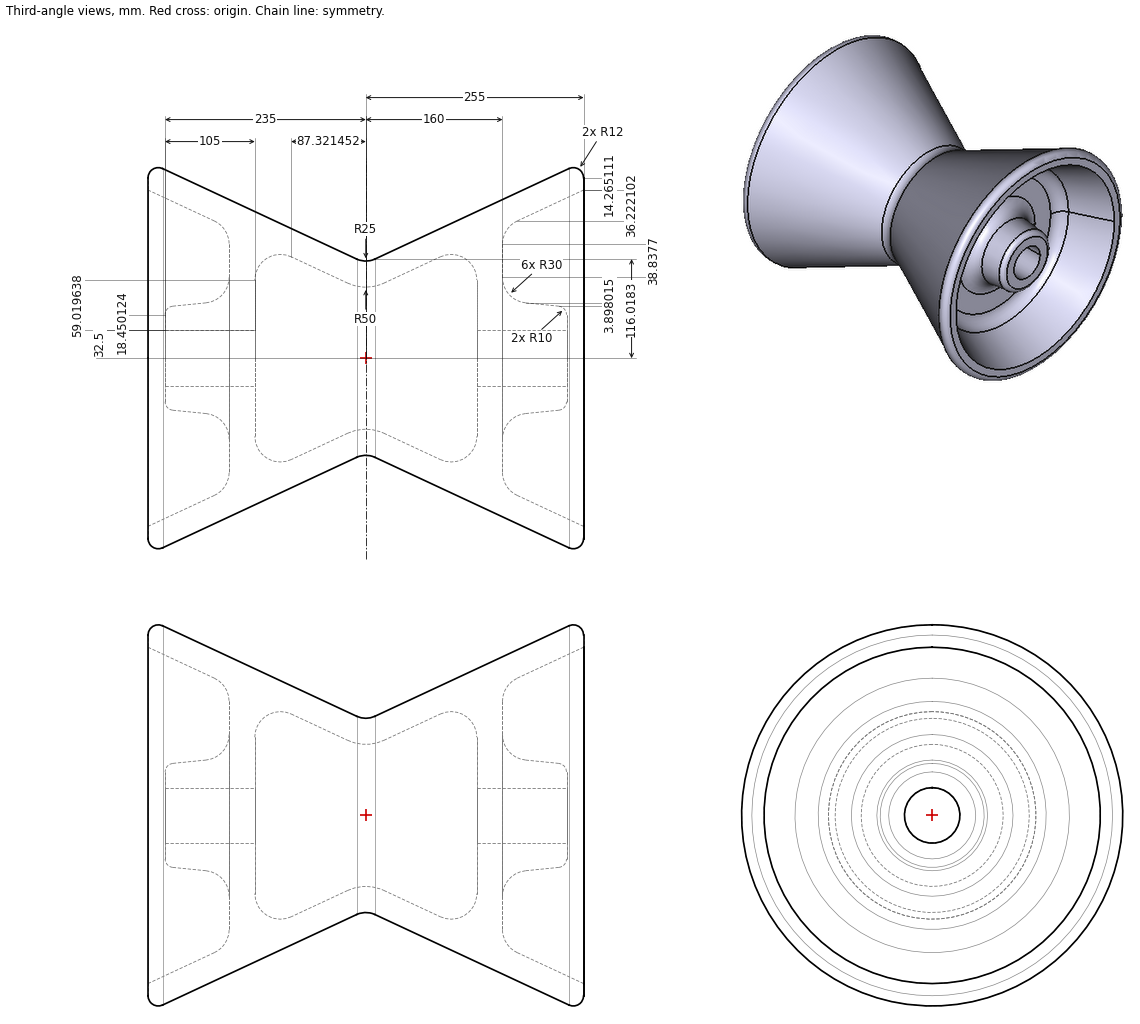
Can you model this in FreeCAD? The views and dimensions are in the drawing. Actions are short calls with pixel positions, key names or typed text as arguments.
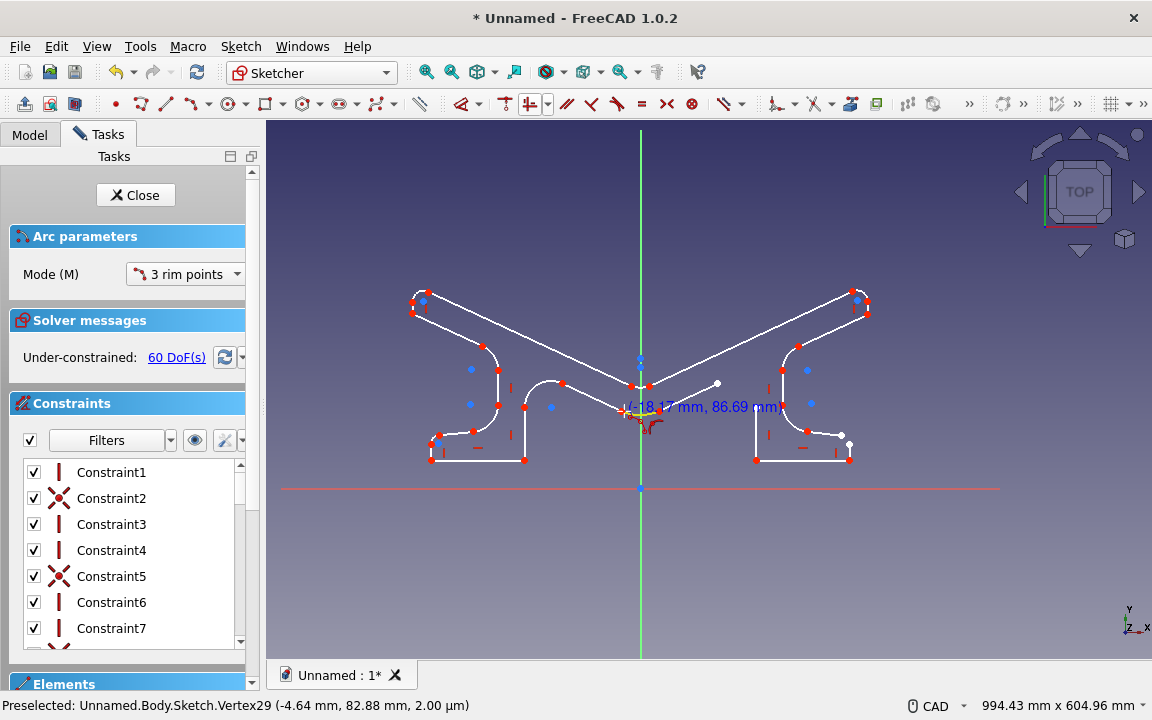
click(718, 384)
click(756, 408)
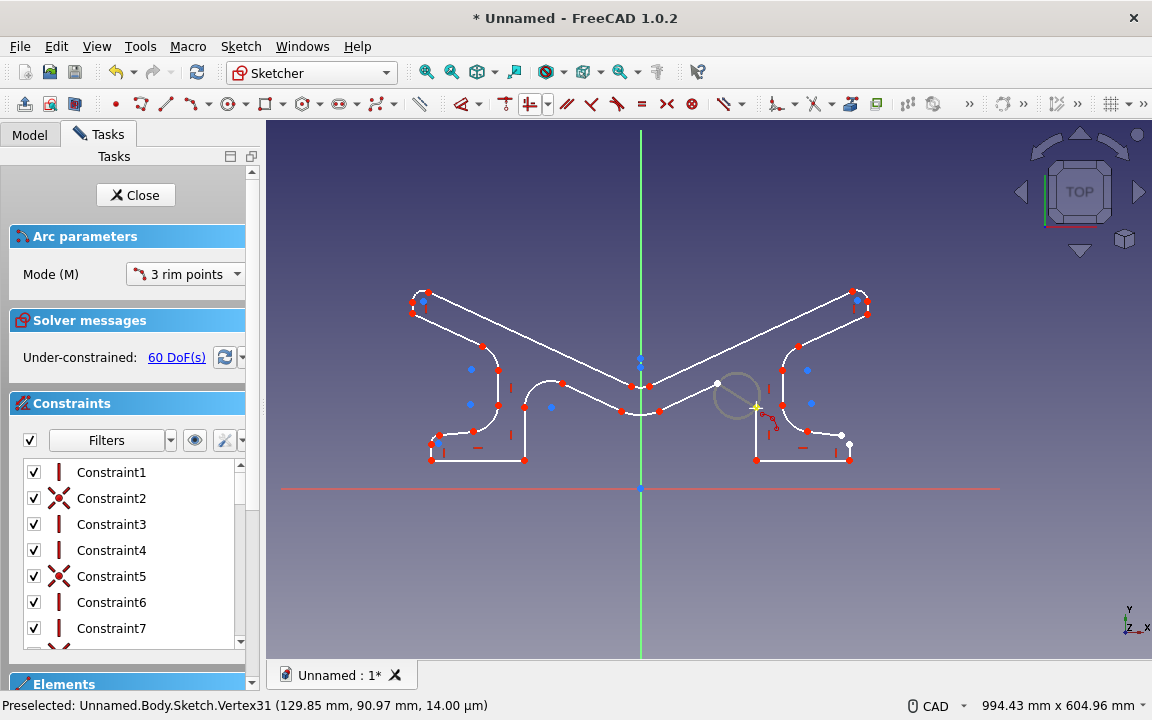
scroll(744, 385, up, 2)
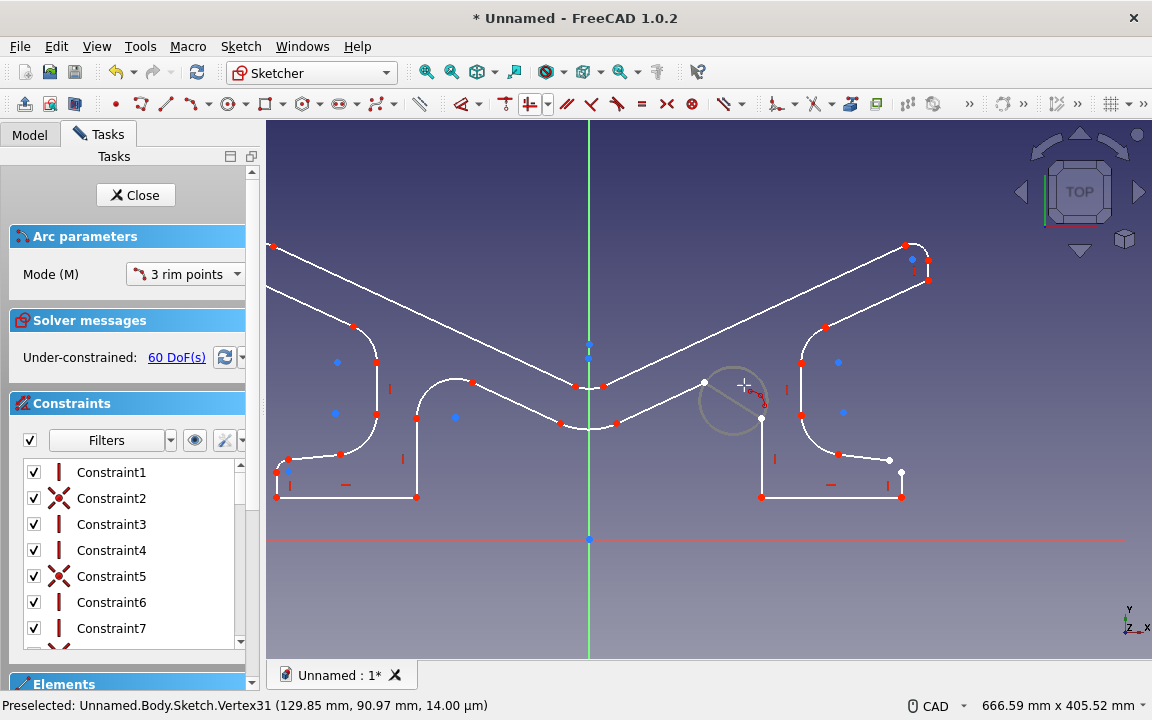
click(744, 384)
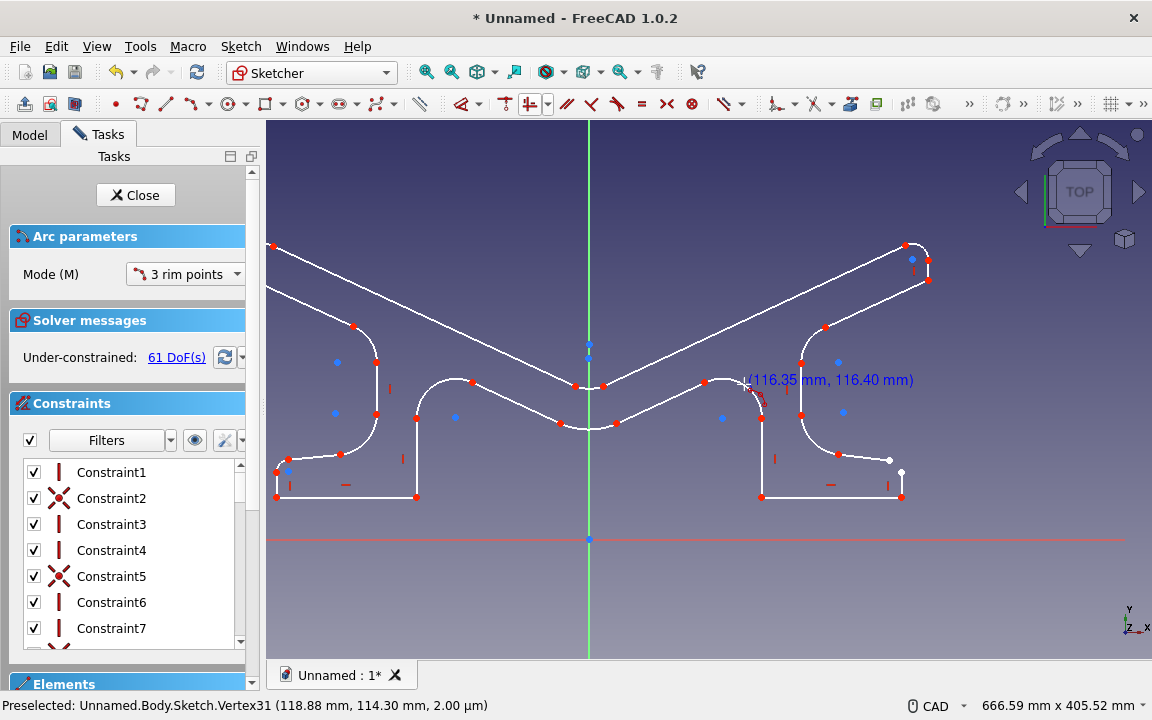
scroll(902, 472, up, 2)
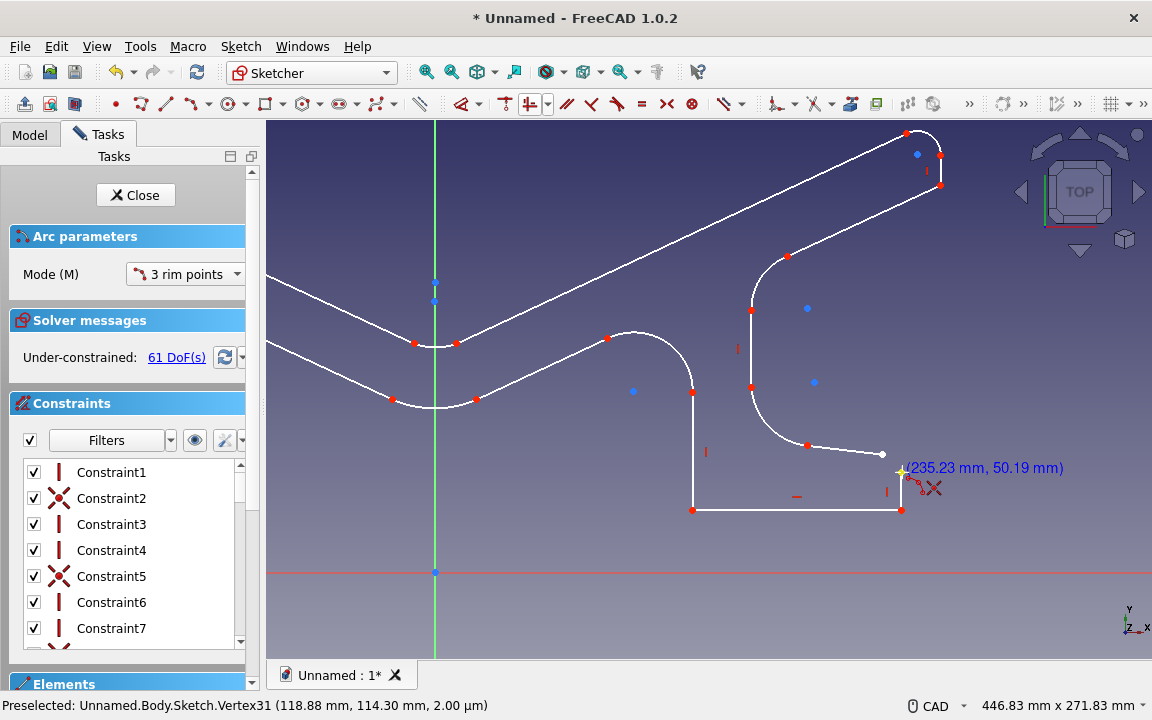
click(901, 473)
click(883, 455)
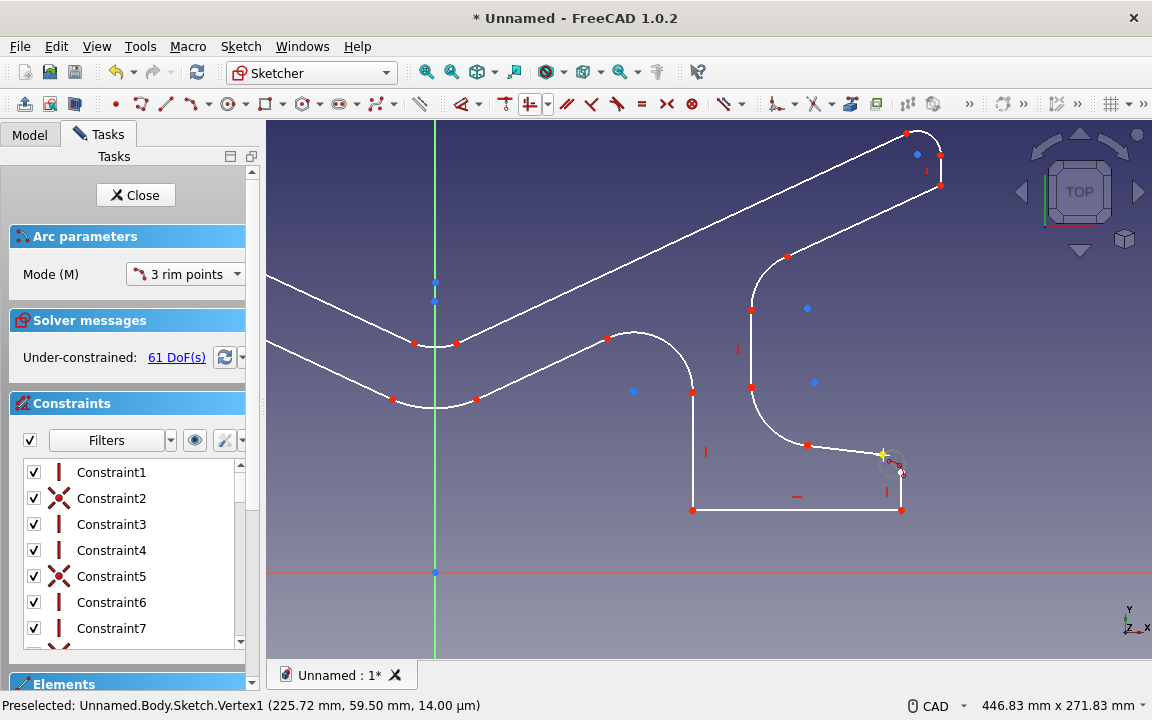
scroll(896, 458, up, 6)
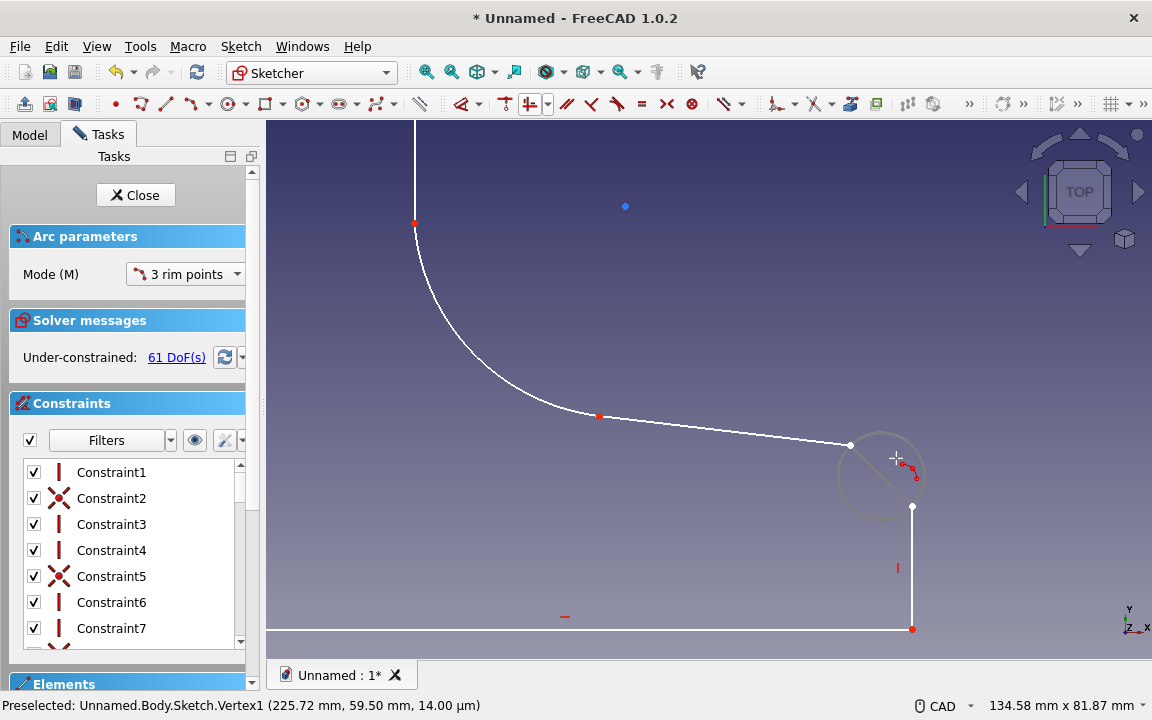
click(895, 458)
key(Escape)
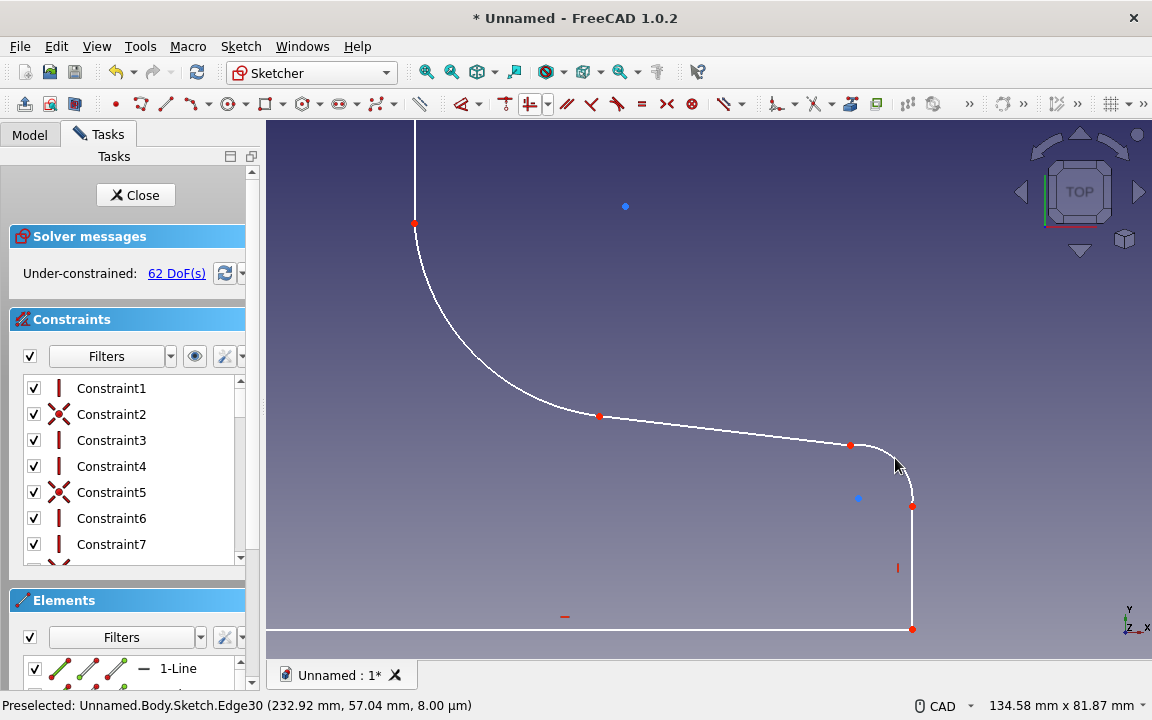
scroll(840, 434, down, 10)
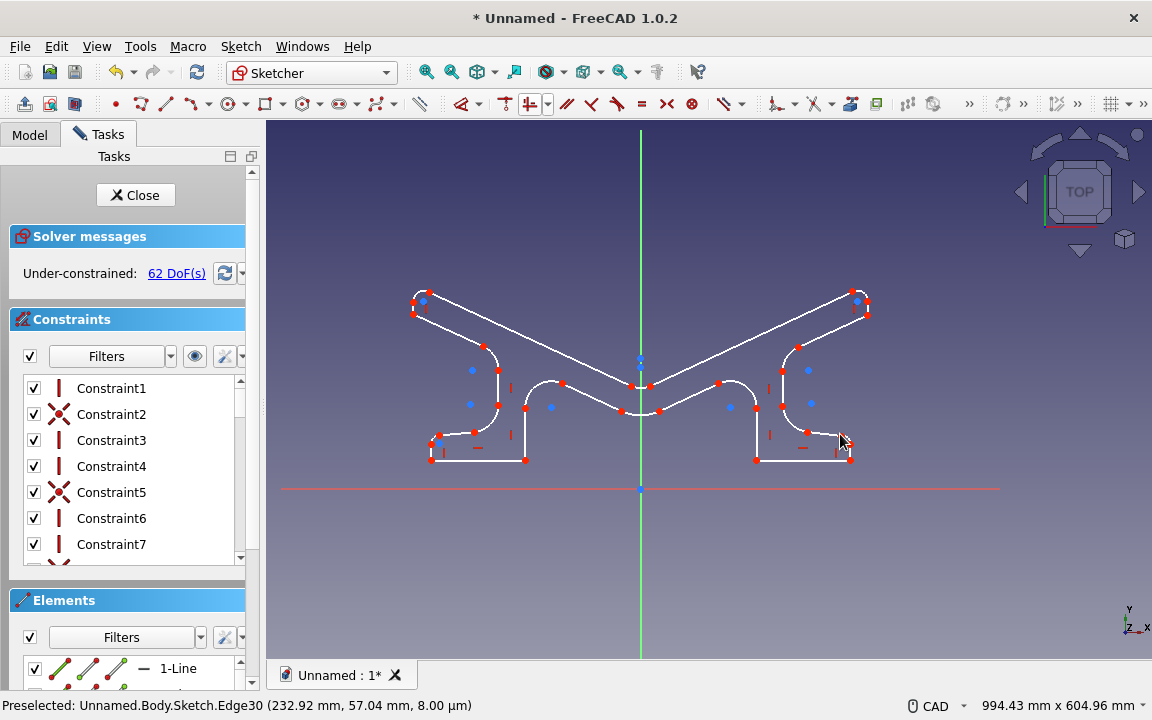
scroll(832, 435, up, 2)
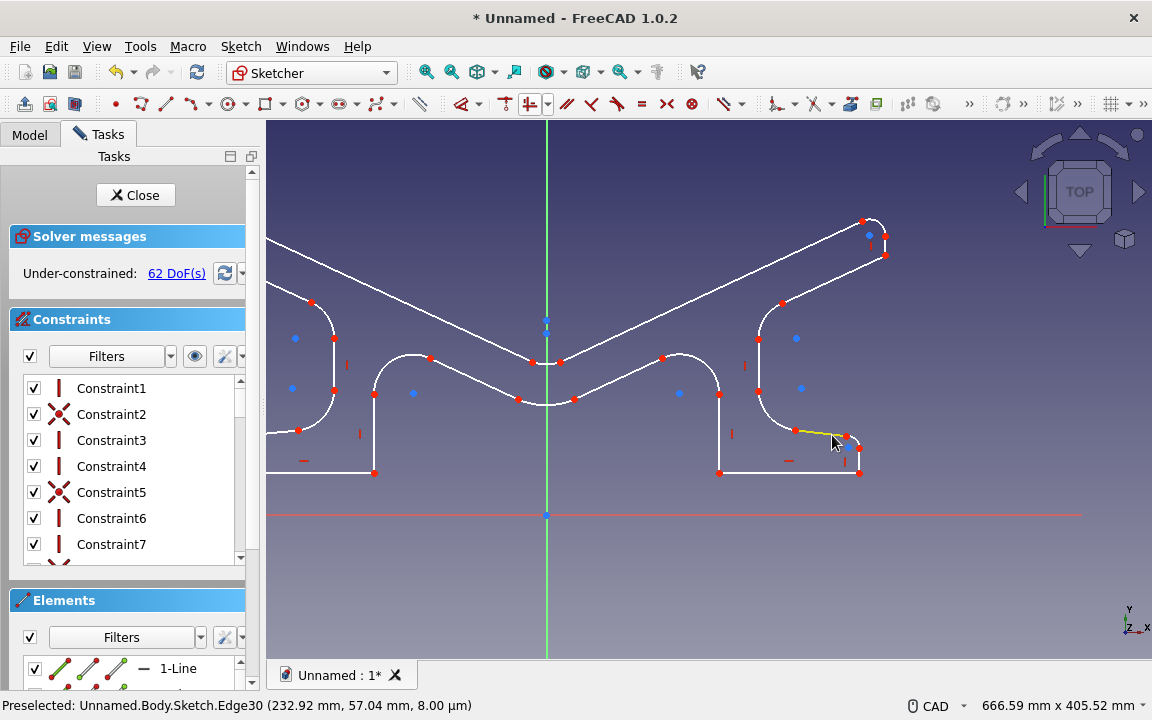
click(831, 435)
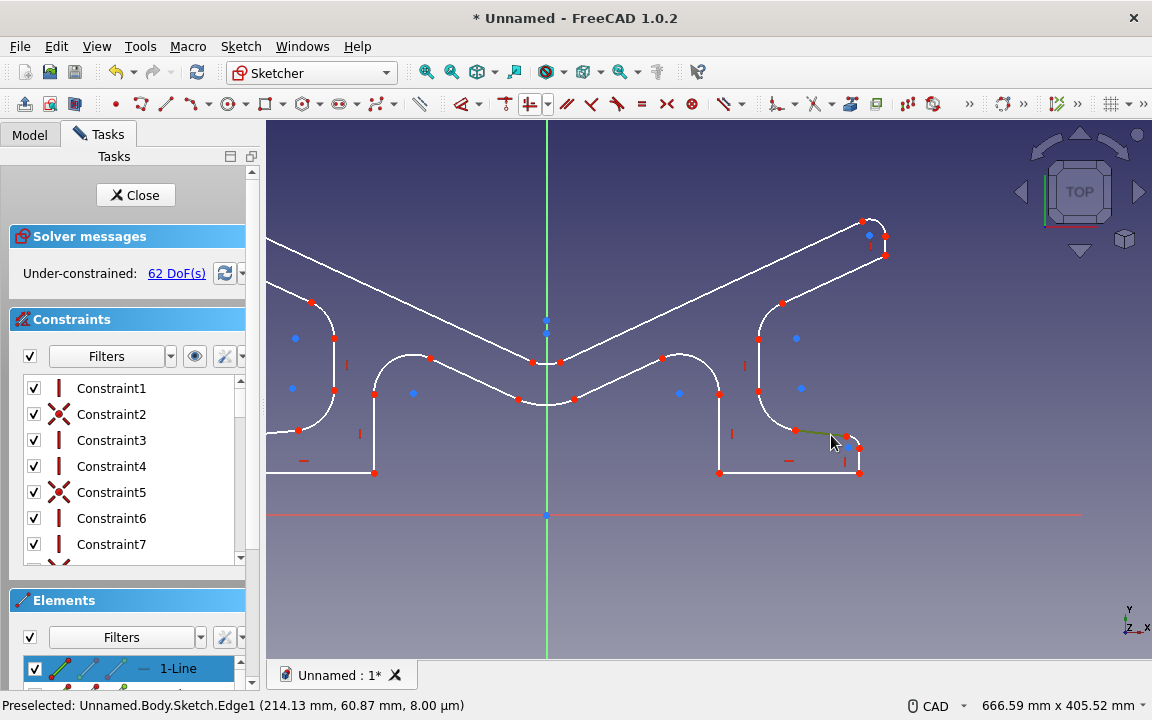
click(763, 408)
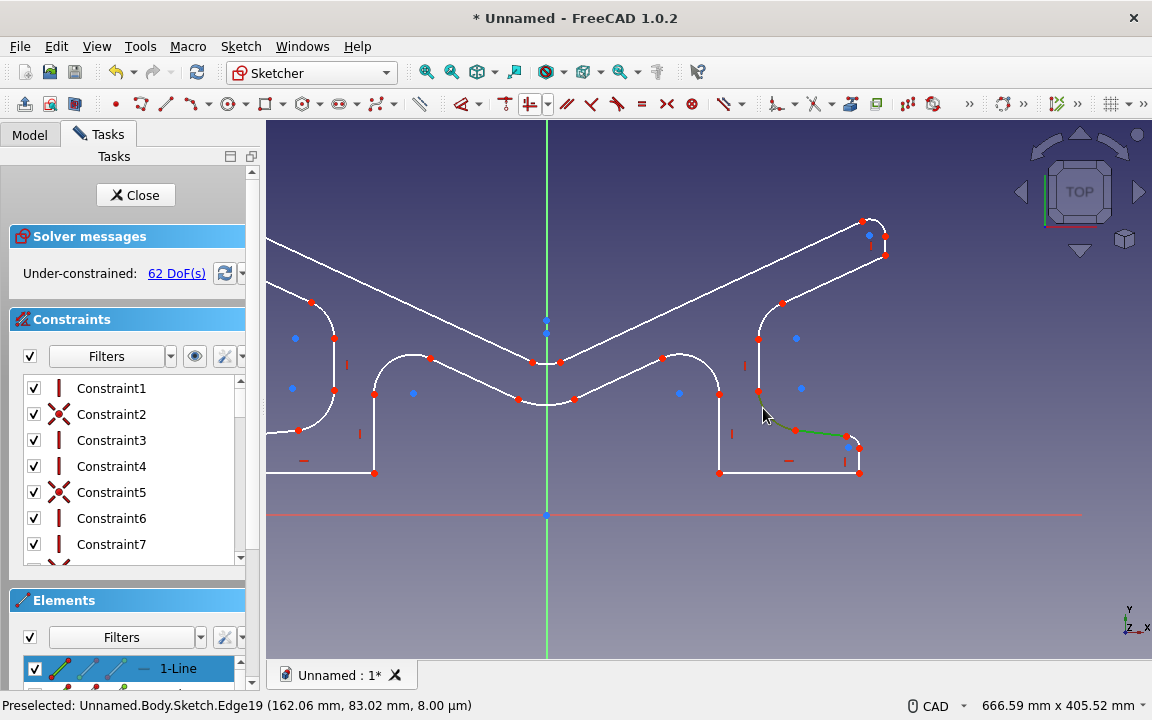
click(617, 104)